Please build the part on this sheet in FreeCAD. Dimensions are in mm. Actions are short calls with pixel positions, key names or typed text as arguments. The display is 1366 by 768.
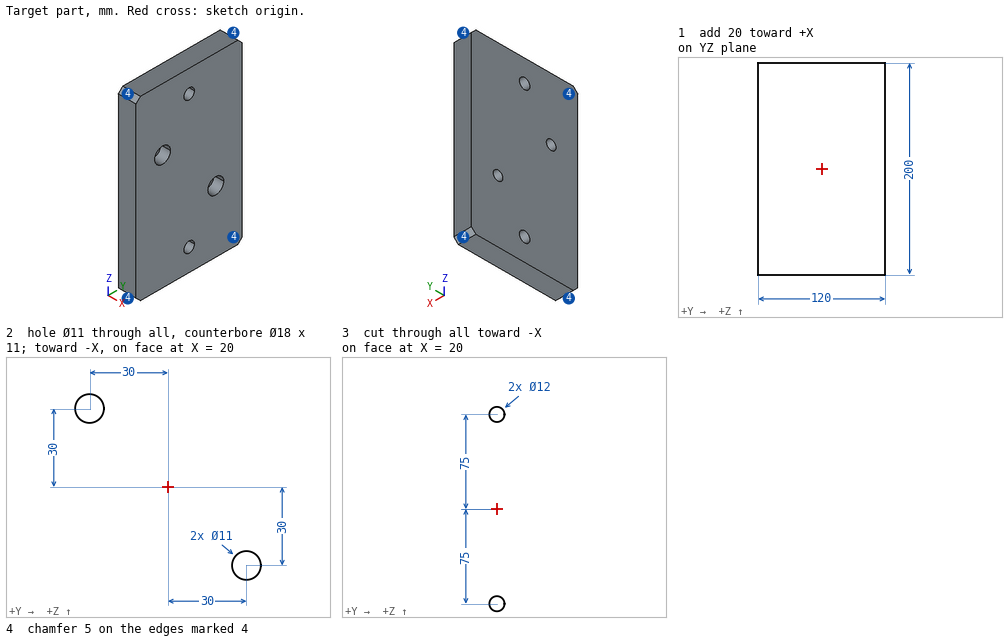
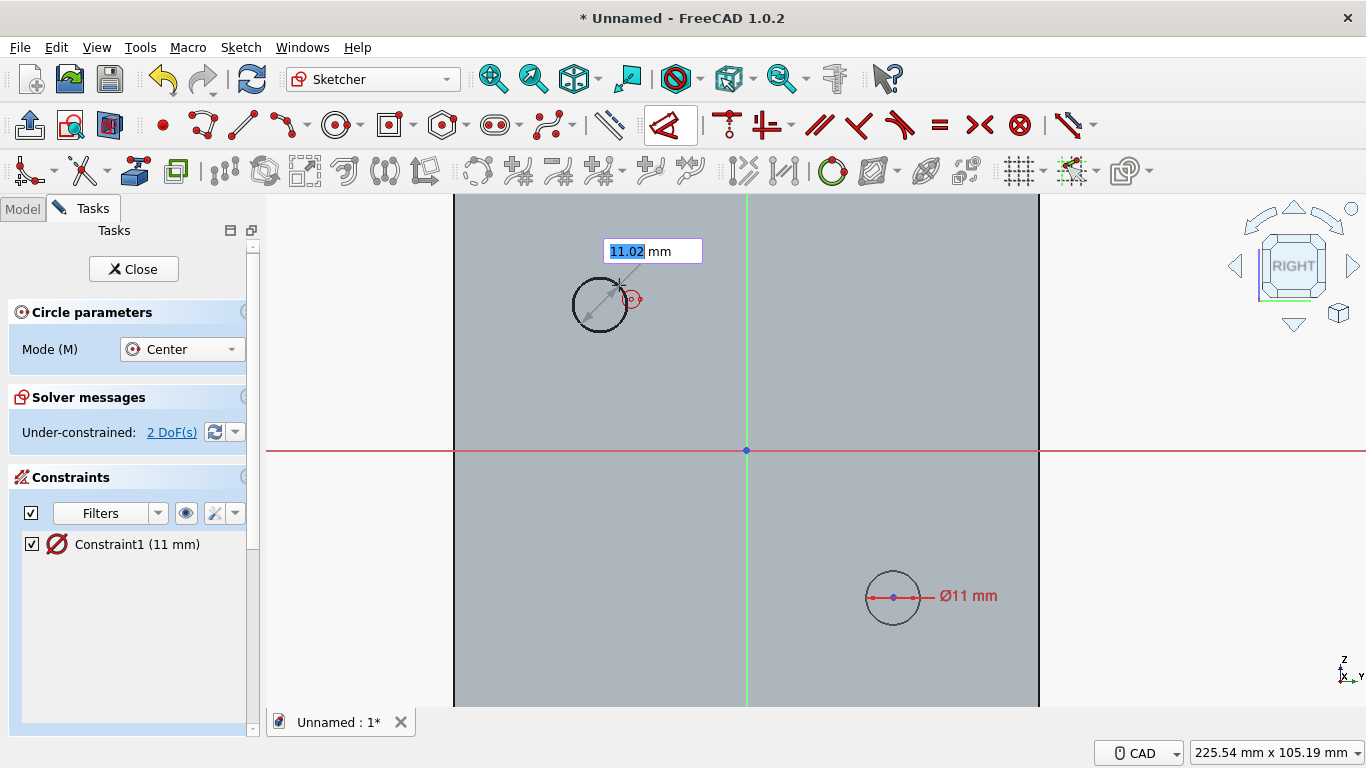
text(11)
key(Return)
key(Escape)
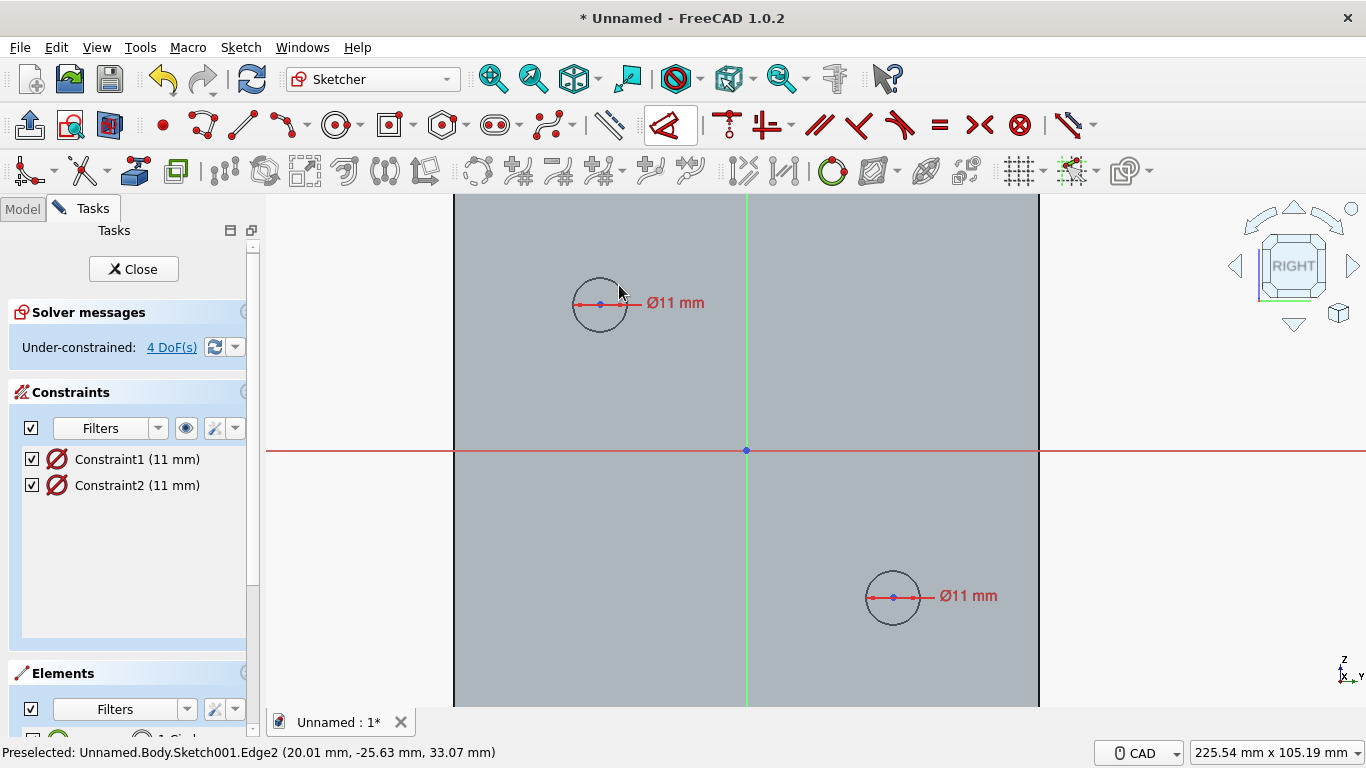
key(d)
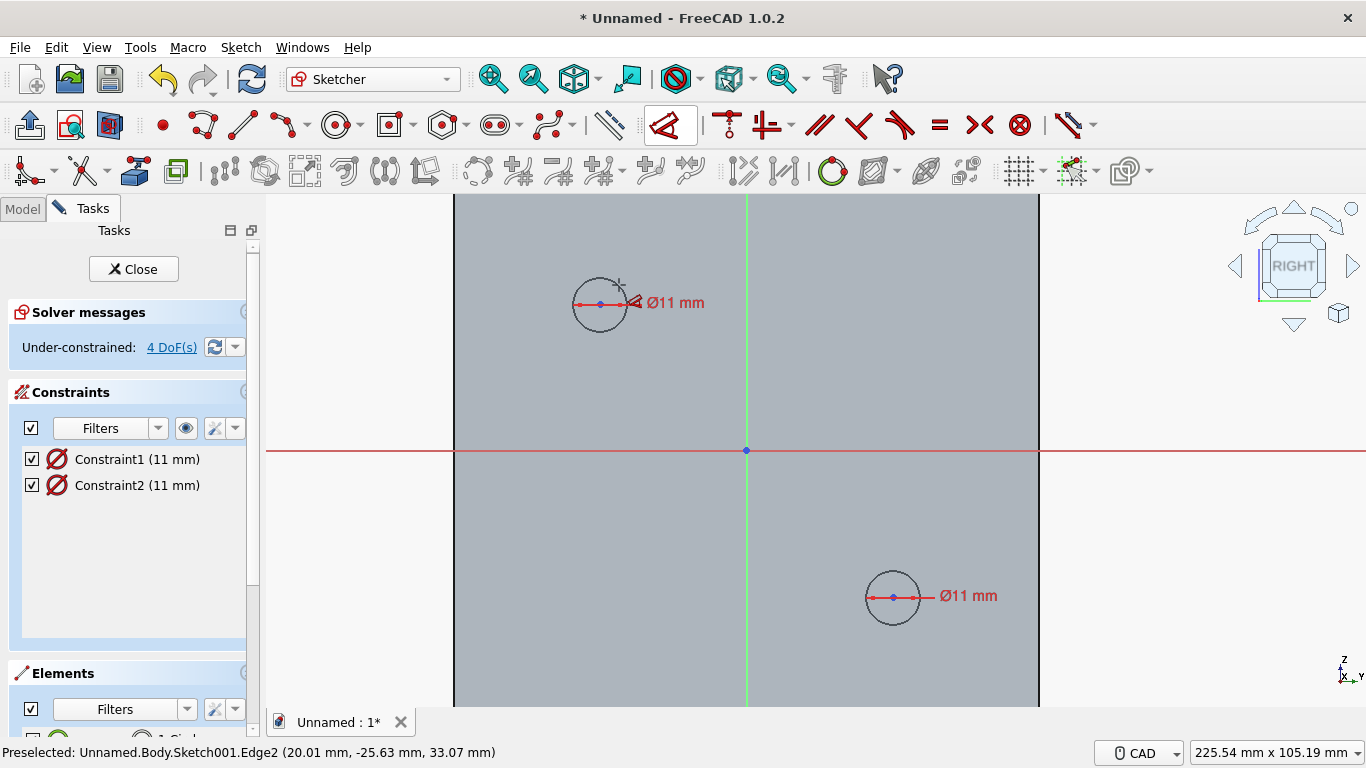
click(893, 598)
click(820, 632)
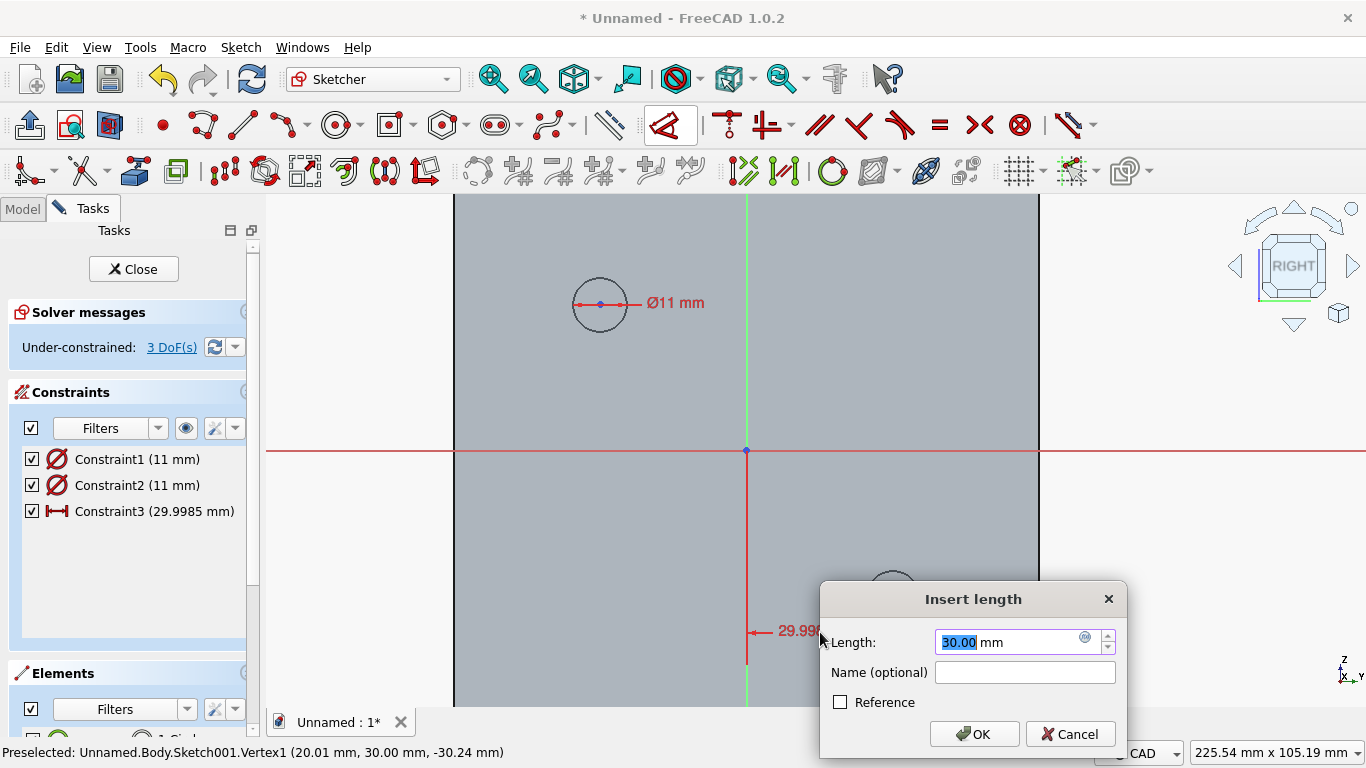
text(30)
key(Return)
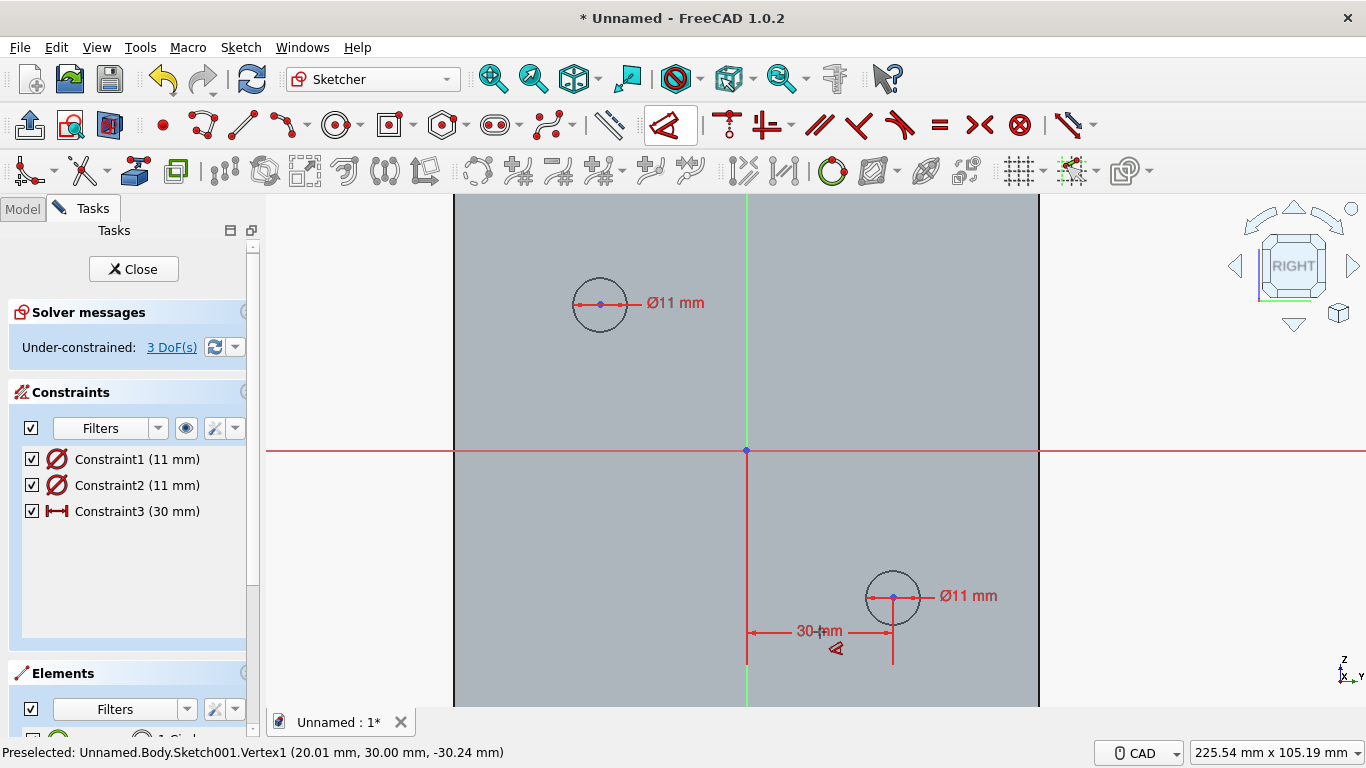
click(893, 598)
click(927, 524)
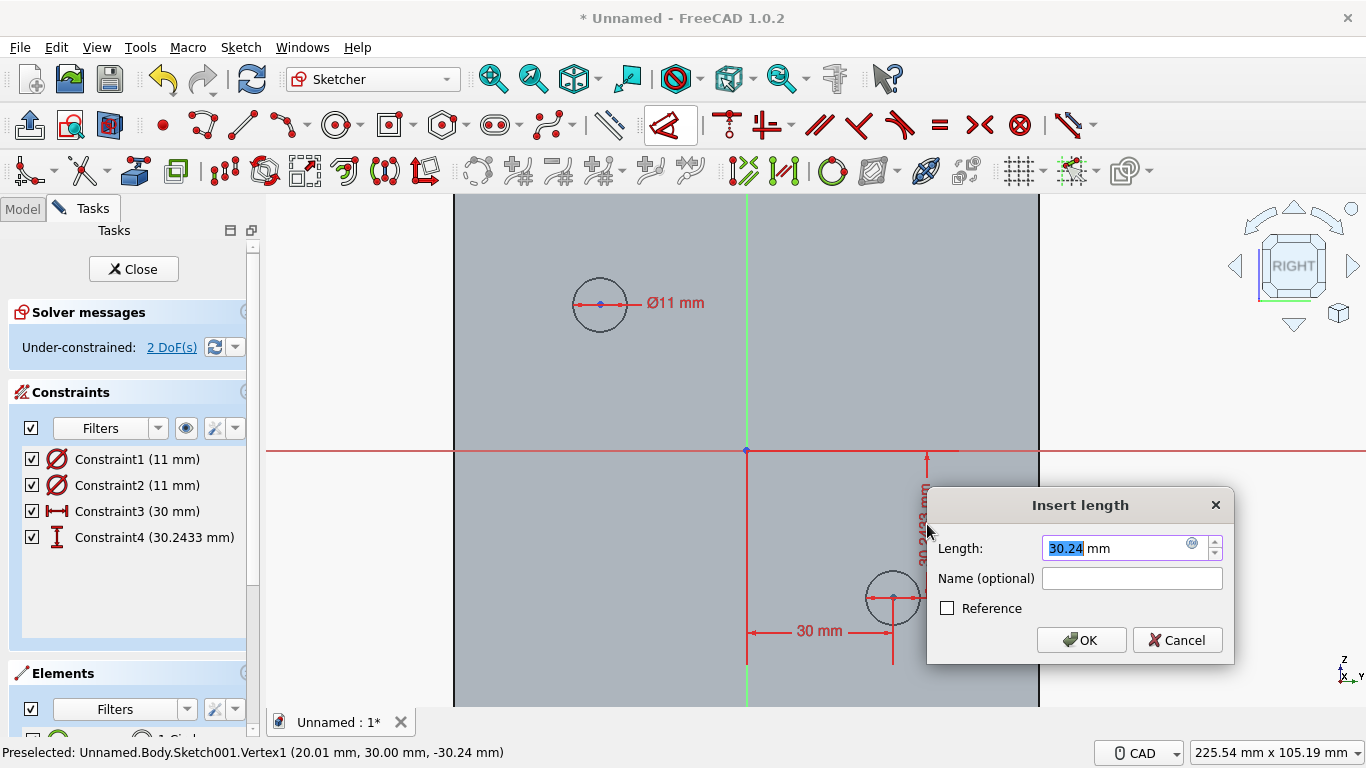
text(30)
key(Return)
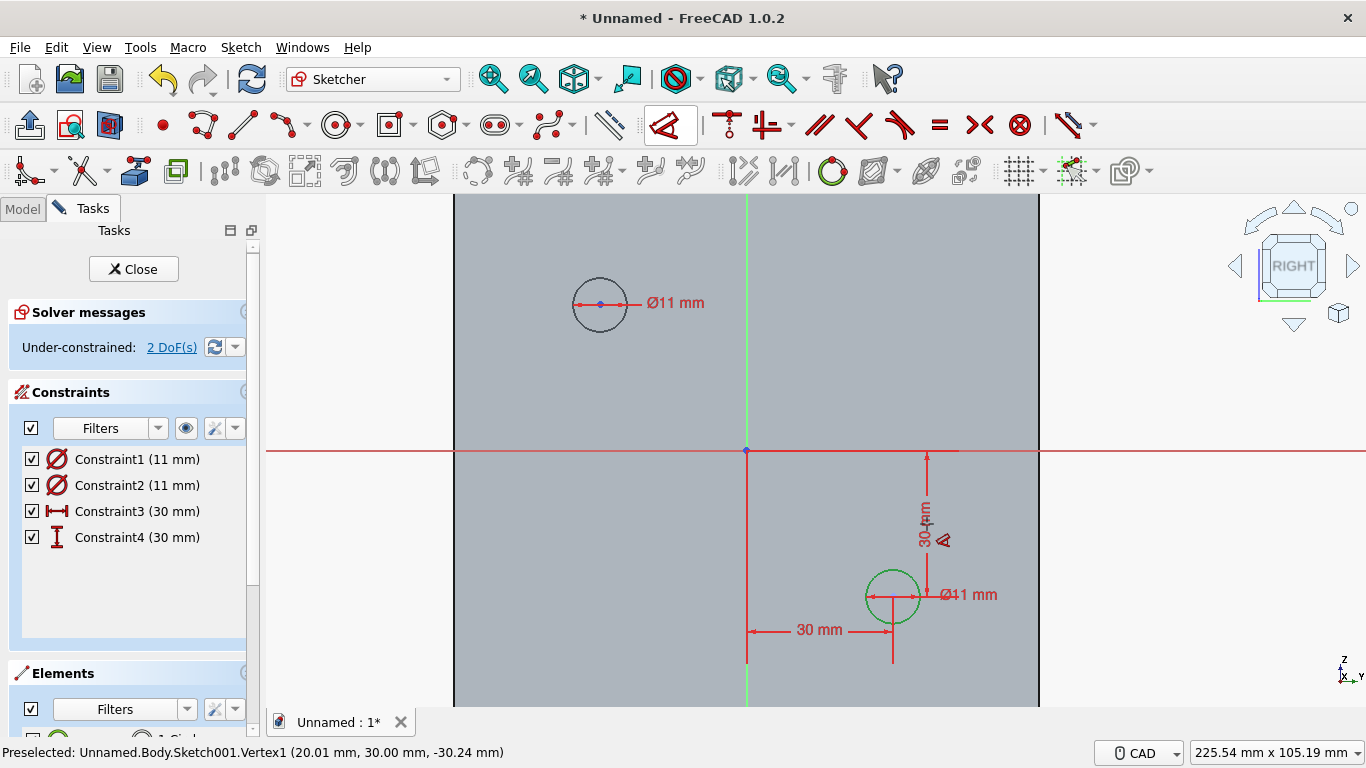
click(600, 305)
click(673, 271)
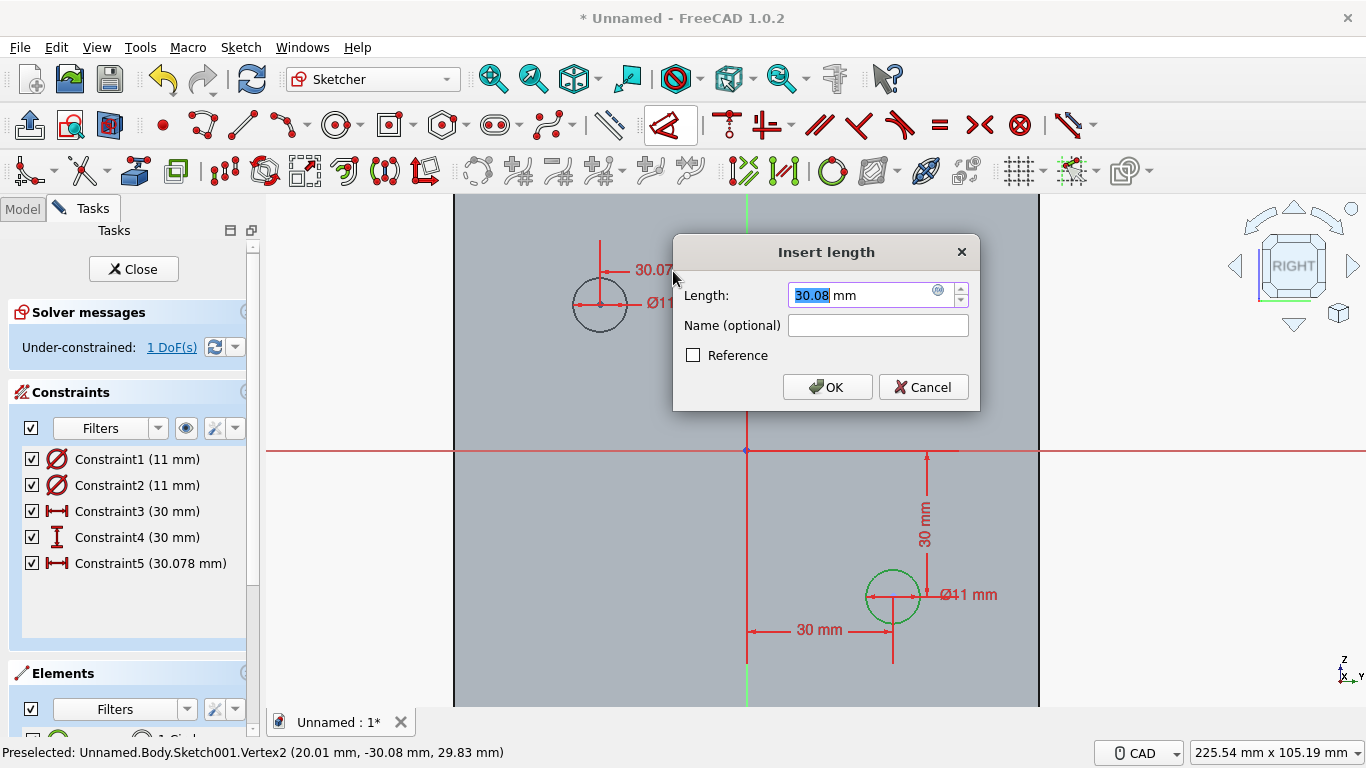
text(30)
key(Return)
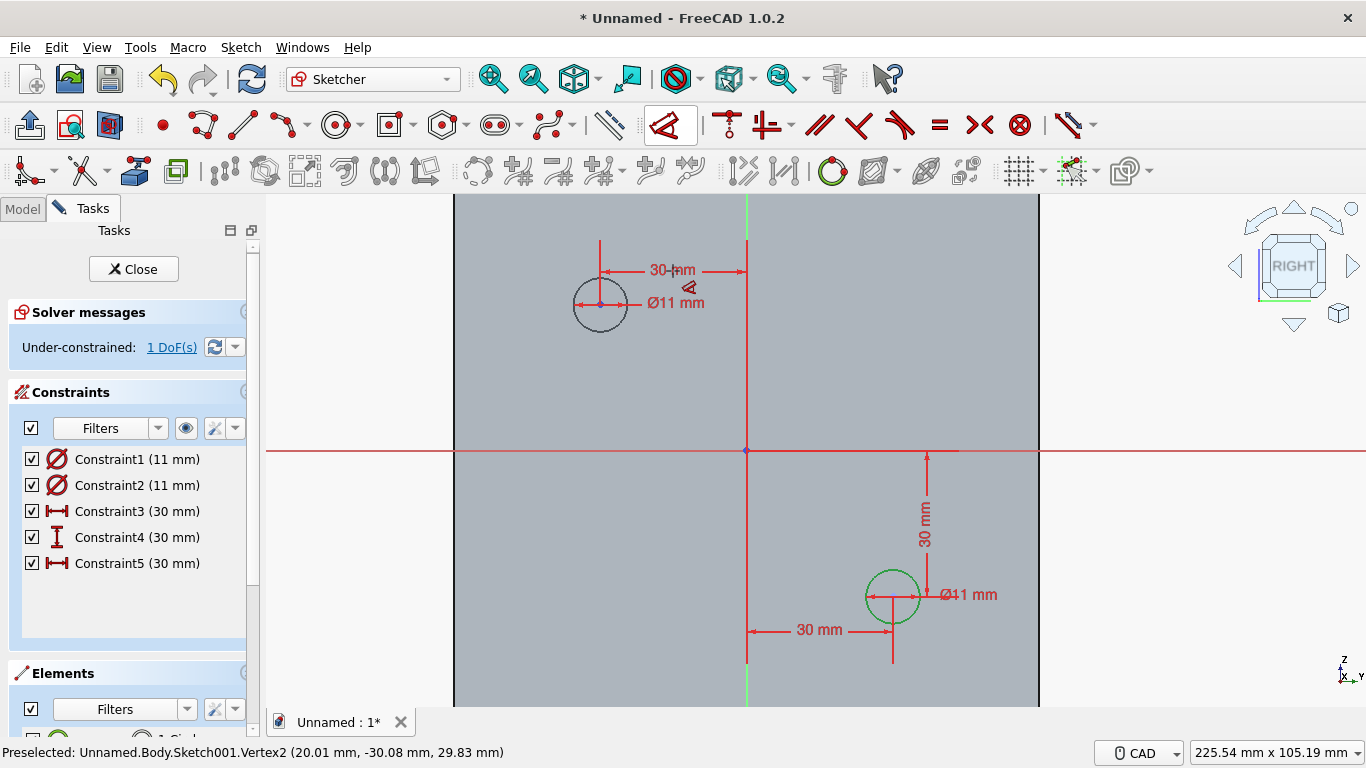
click(600, 305)
click(566, 378)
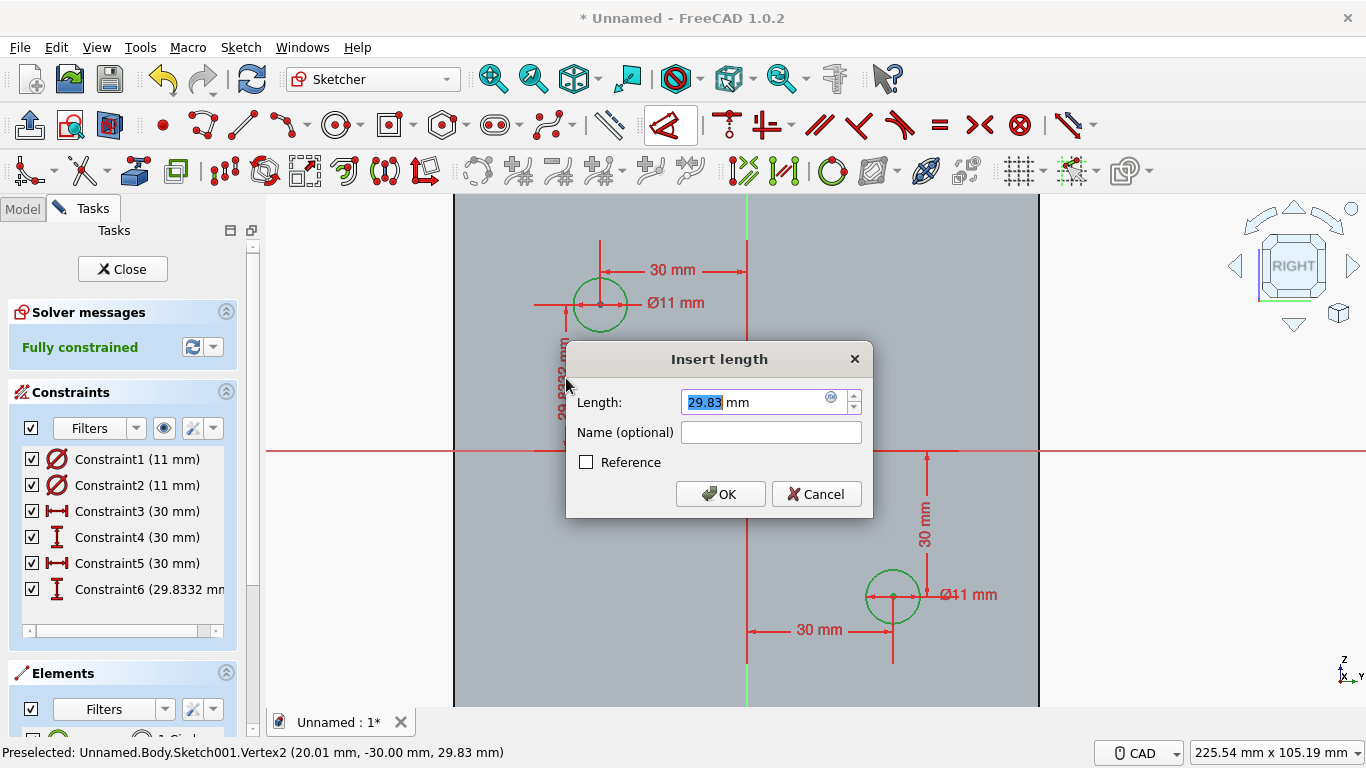
text(30)
key(Return)
key(Escape)